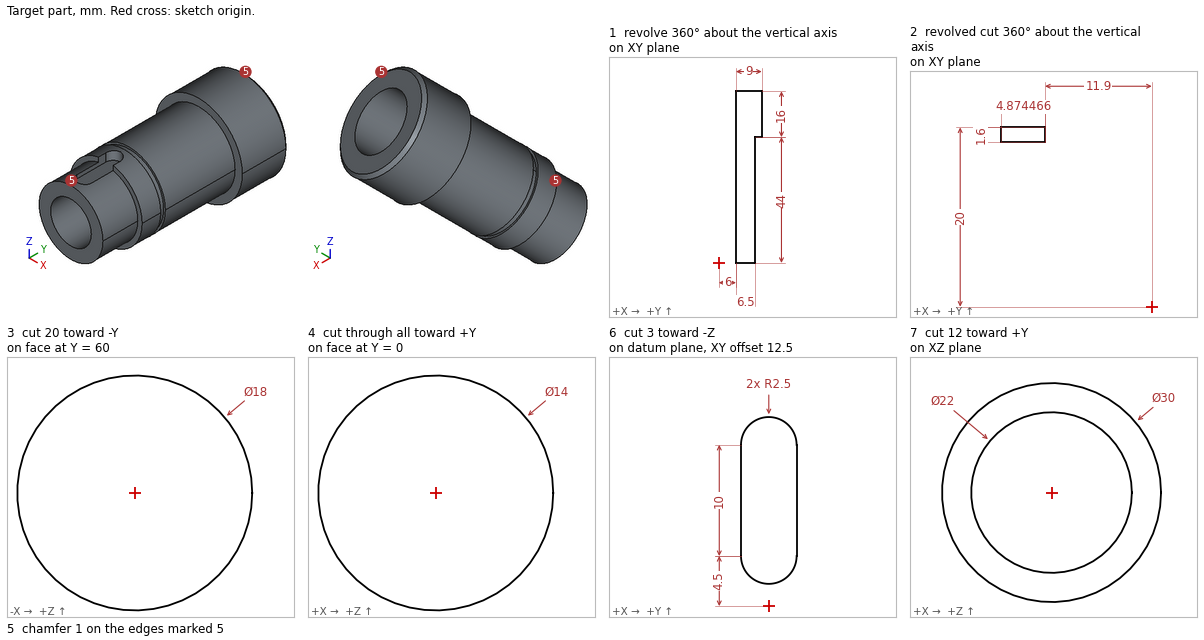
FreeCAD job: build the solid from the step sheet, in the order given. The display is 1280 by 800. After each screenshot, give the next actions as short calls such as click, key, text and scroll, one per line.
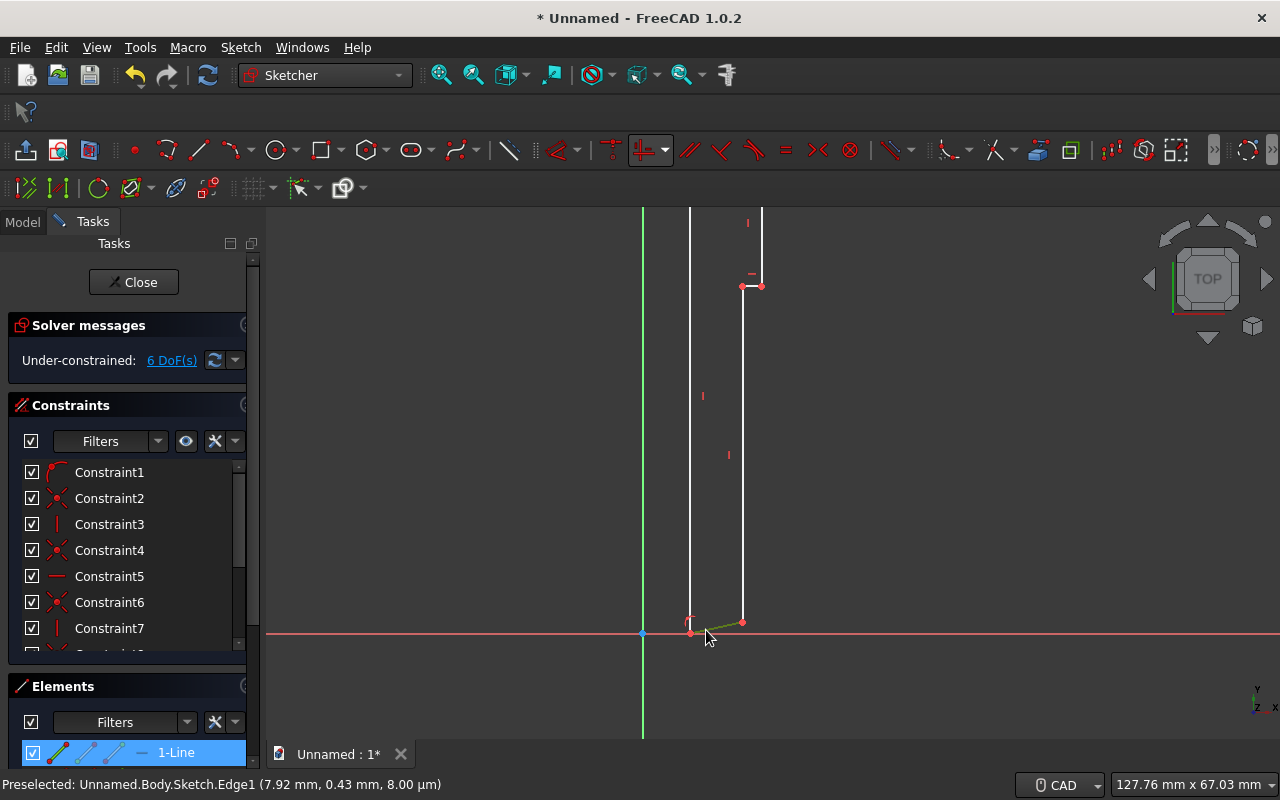
click(668, 150)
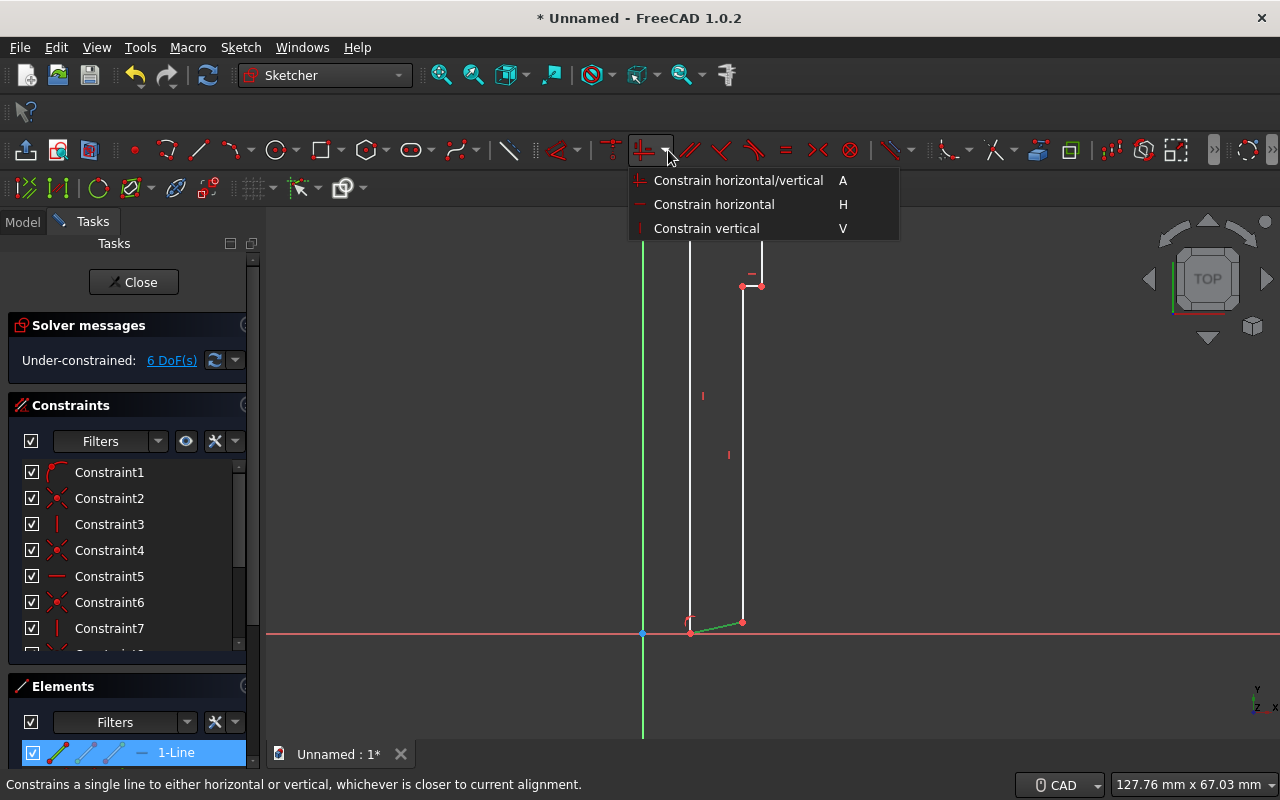
click(764, 204)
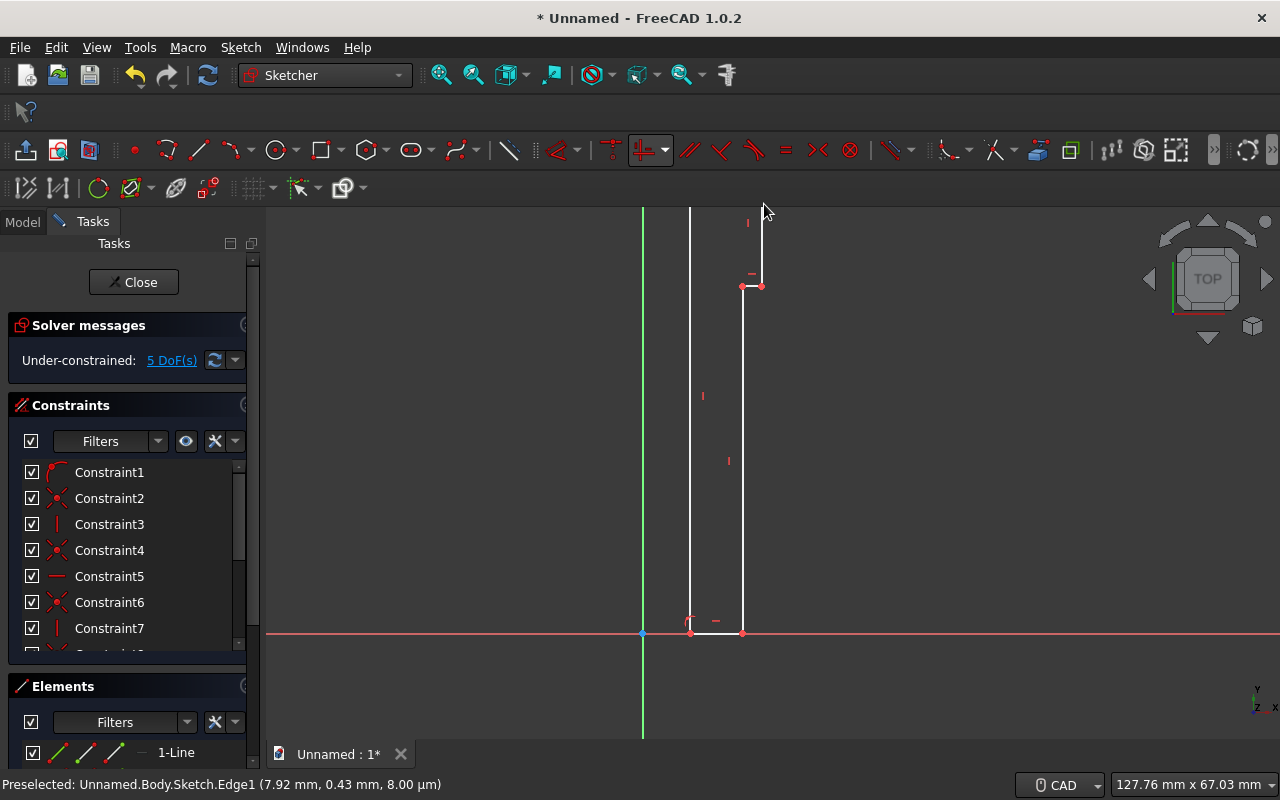
click(556, 150)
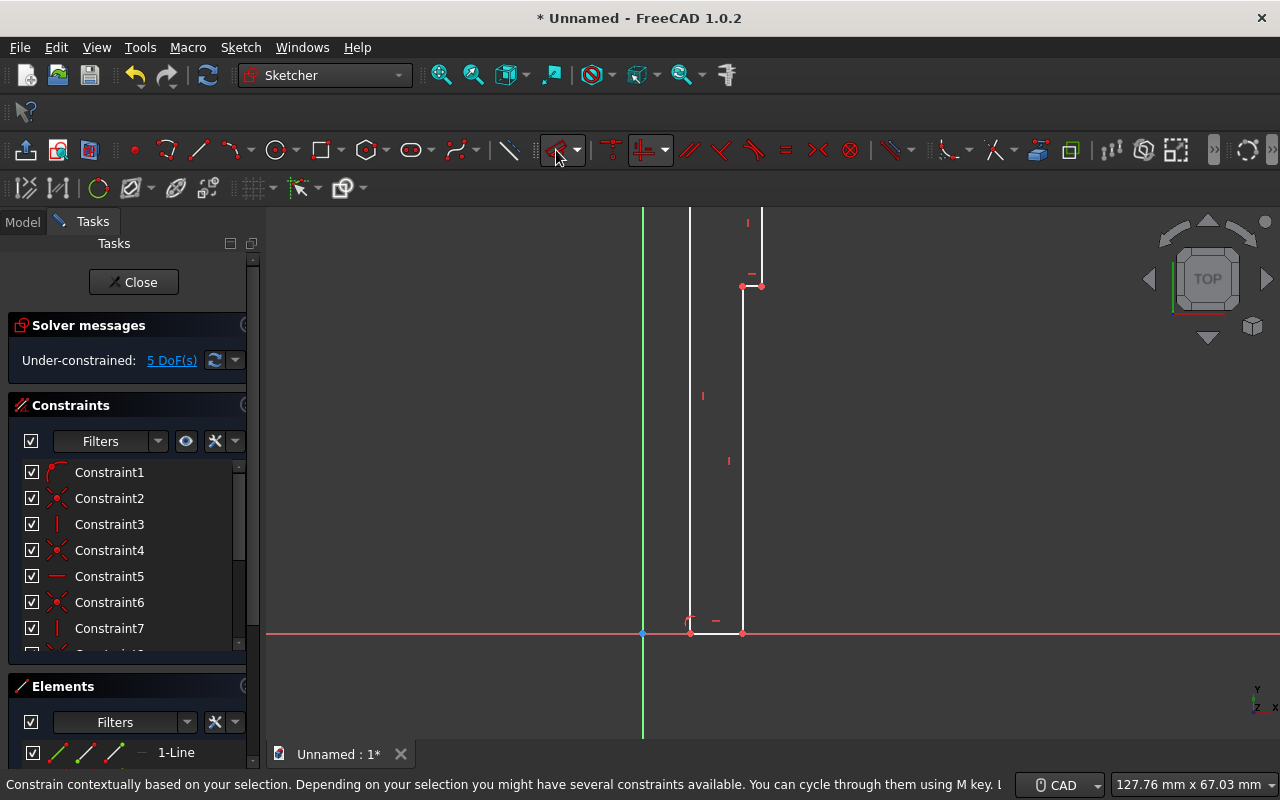
scroll(709, 631, down, 2)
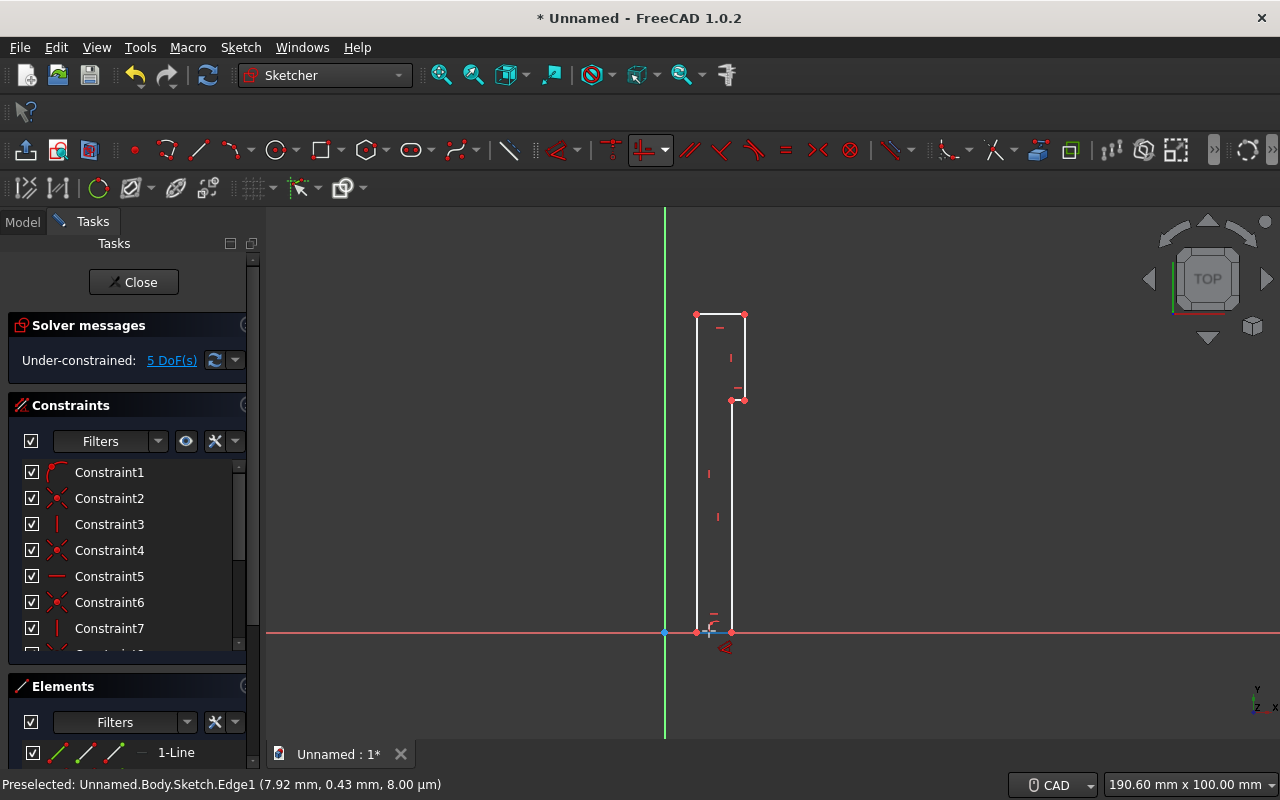
click(730, 314)
click(721, 280)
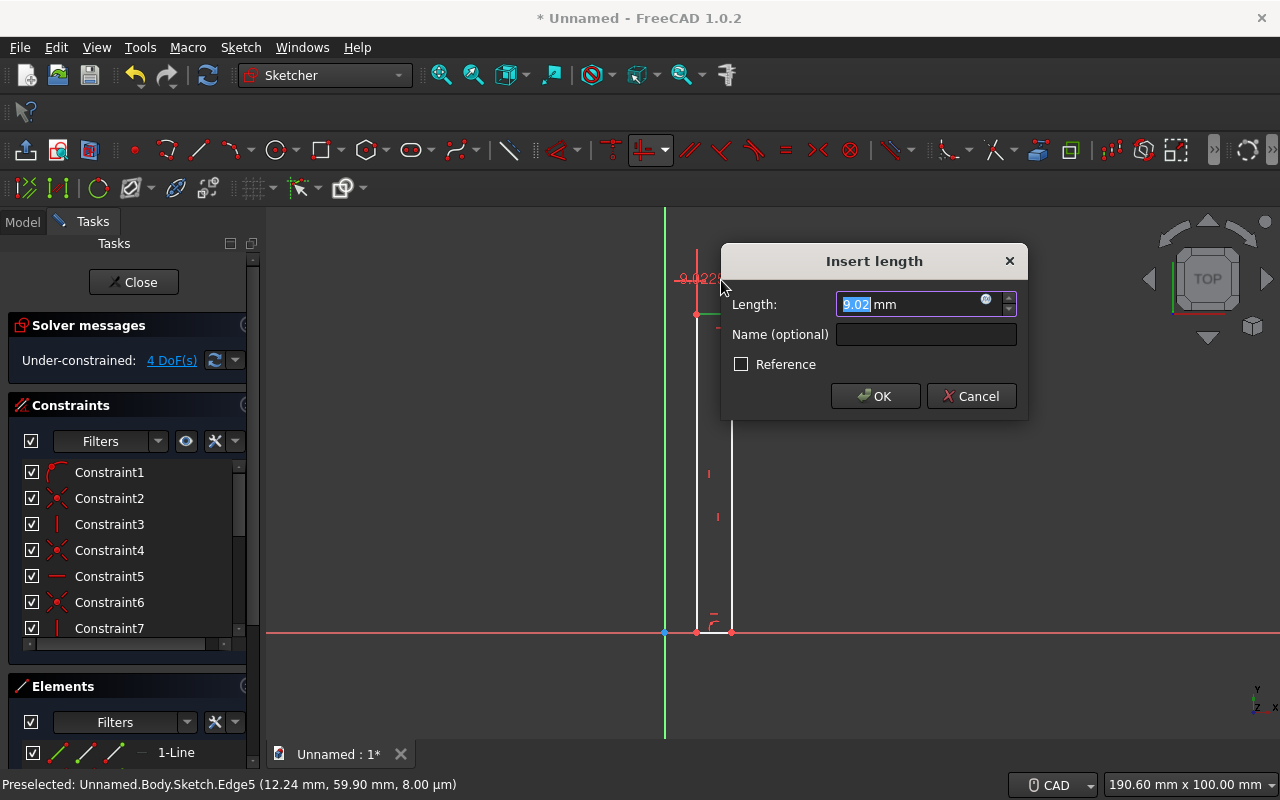
text(9)
key(Return)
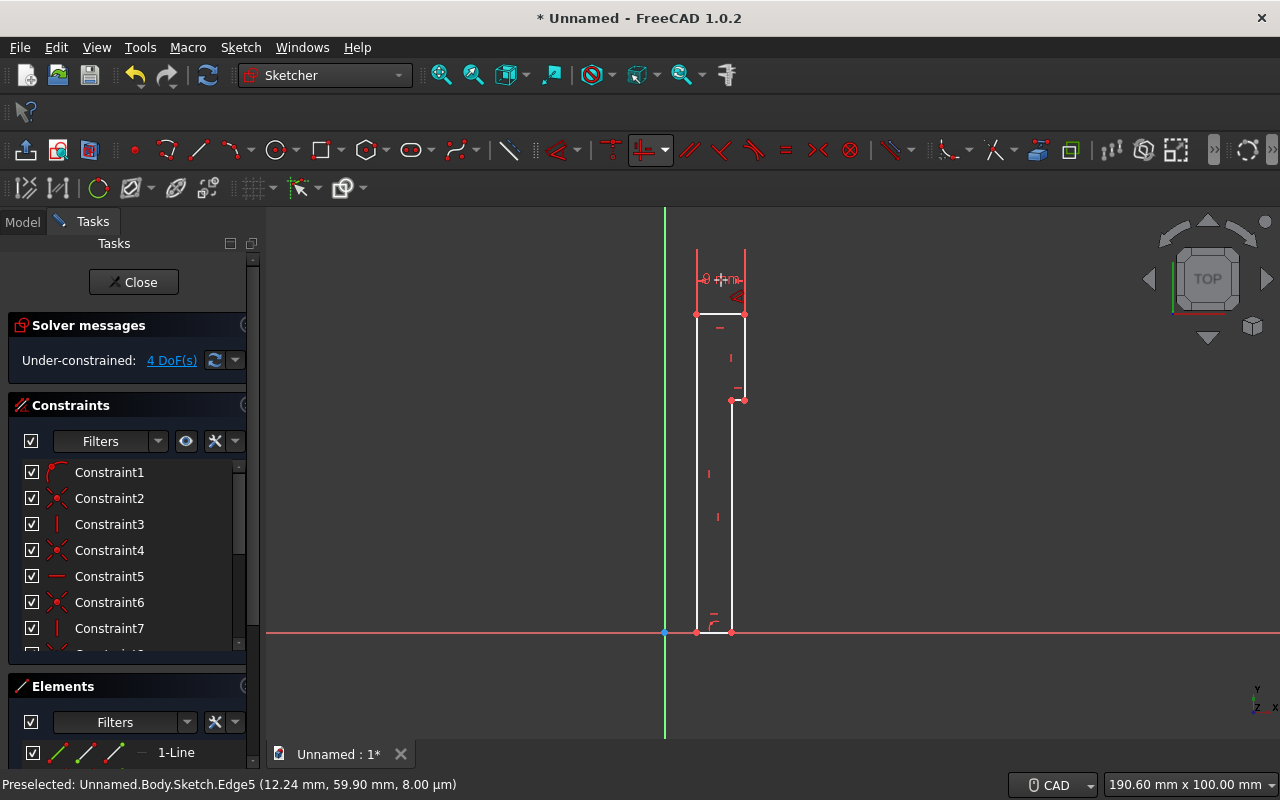
click(732, 563)
click(766, 517)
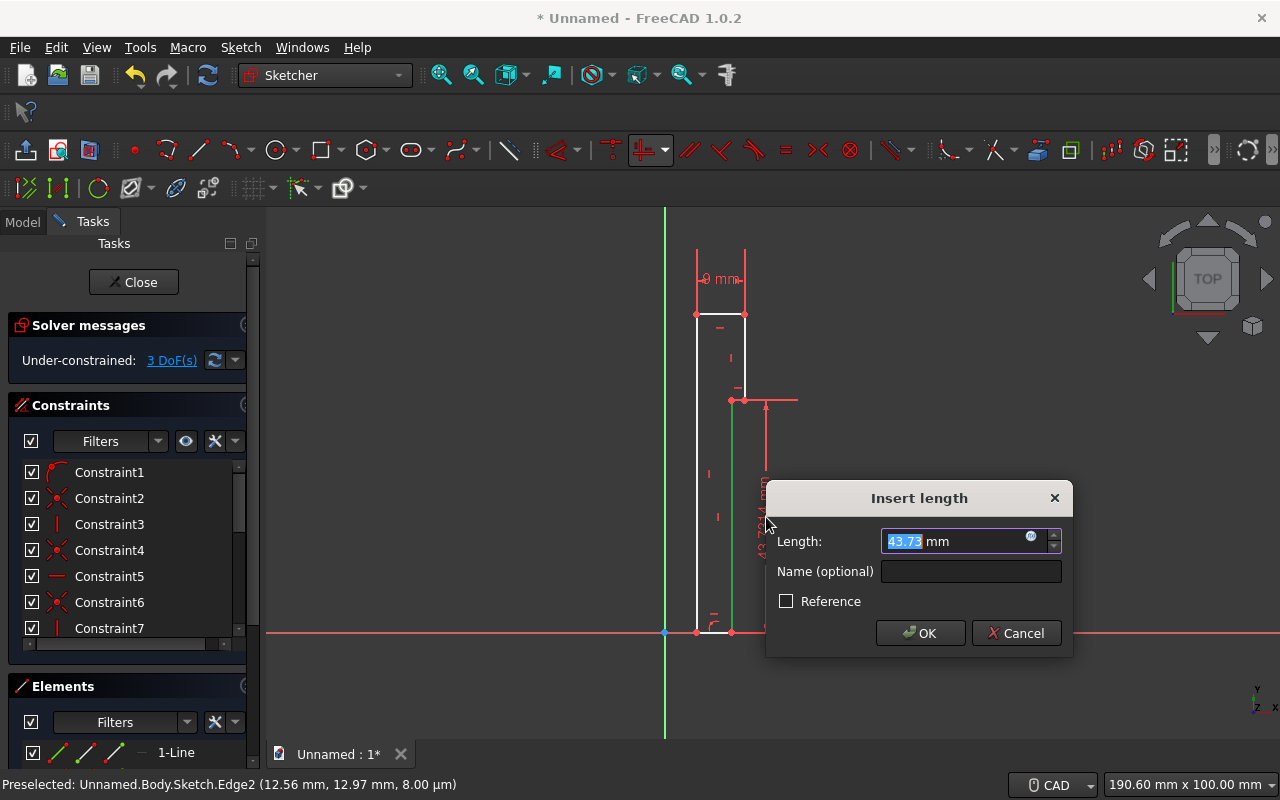
text(44)
key(Return)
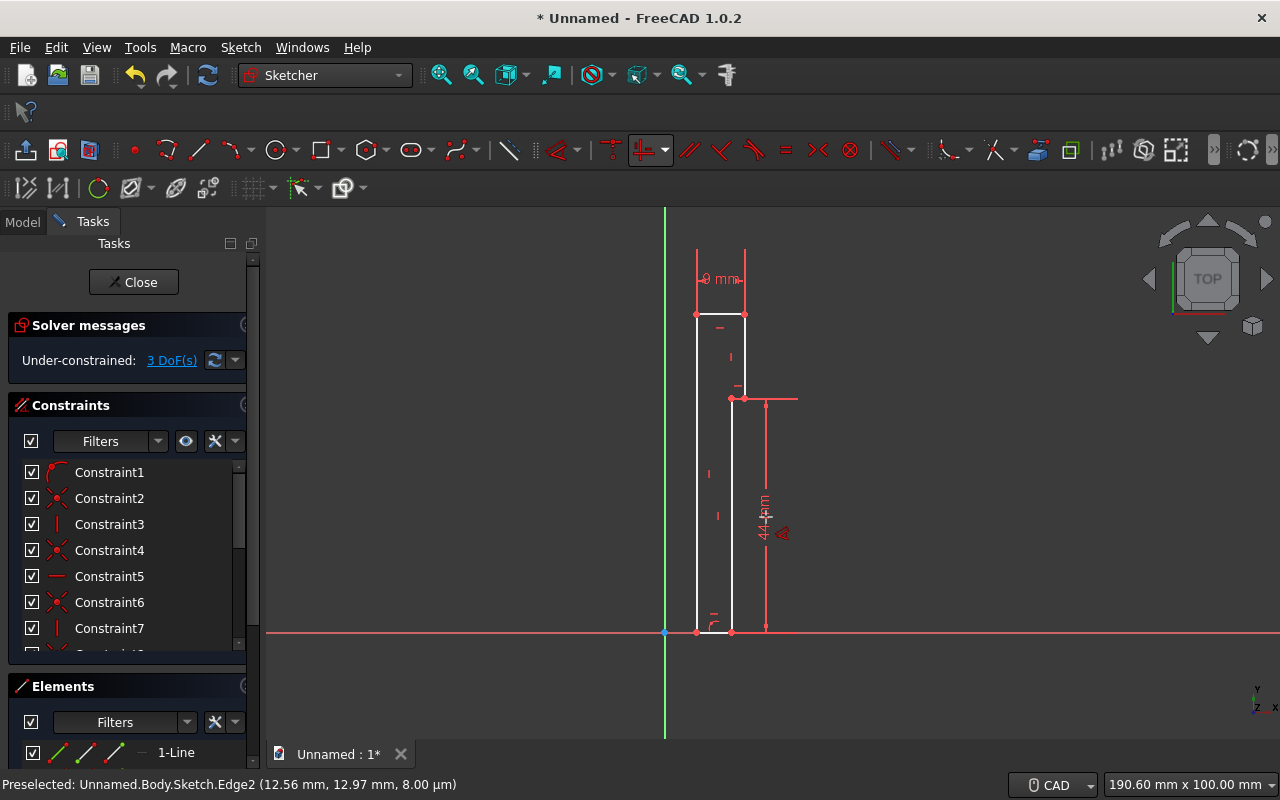
click(745, 374)
click(779, 357)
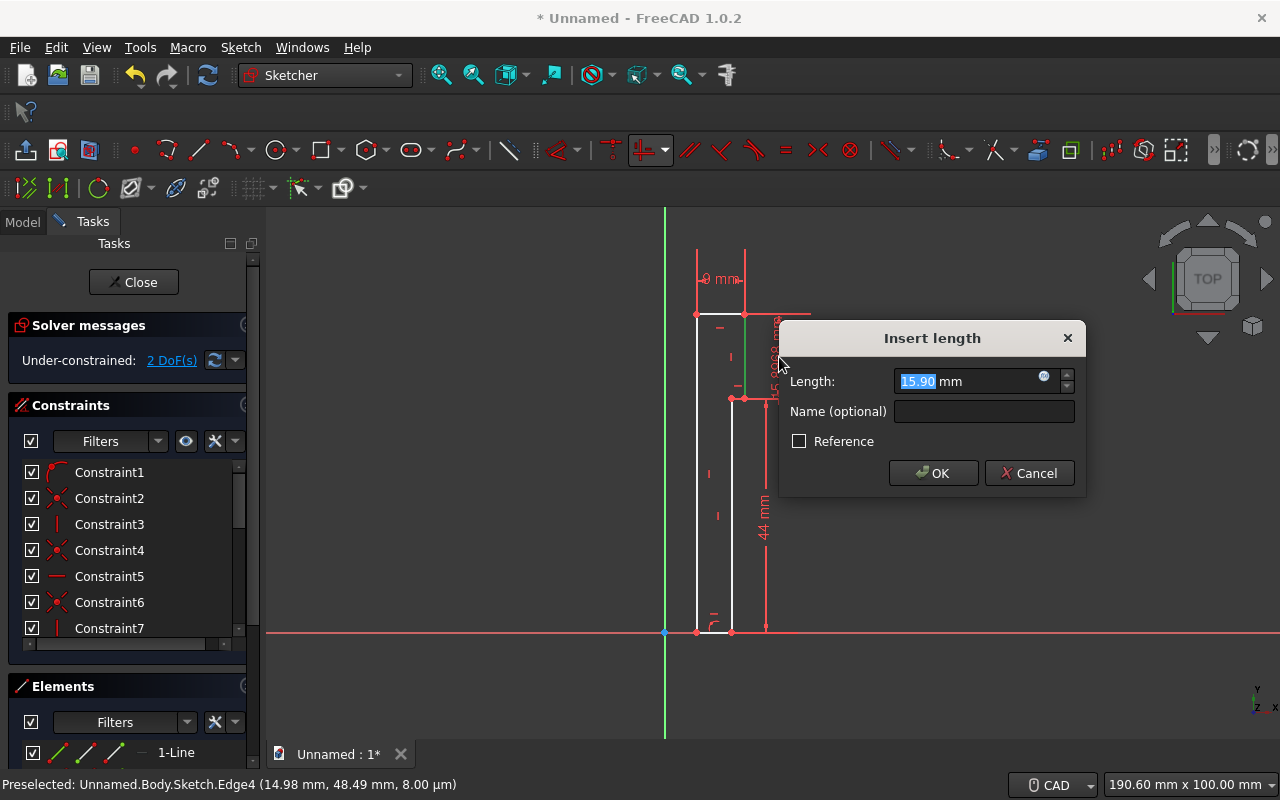
text(16)
key(Return)